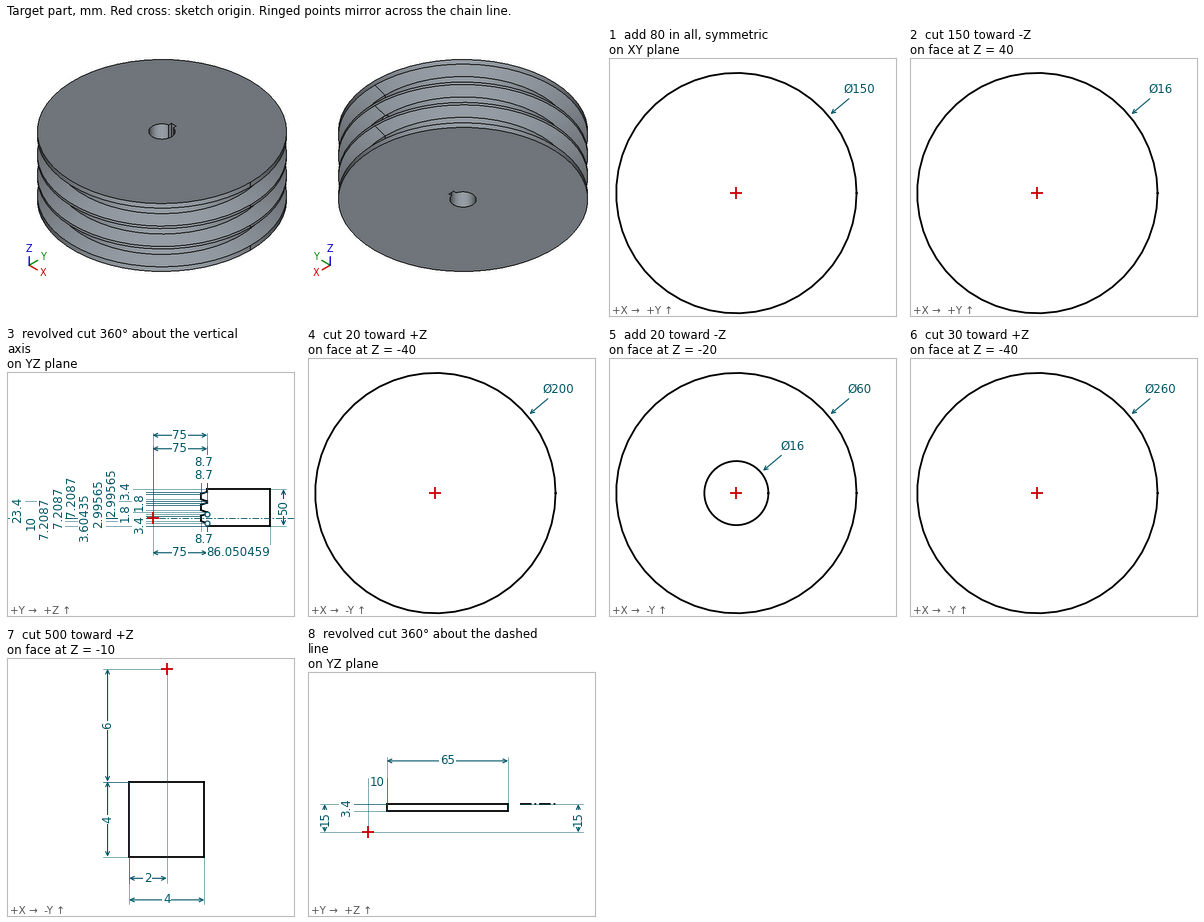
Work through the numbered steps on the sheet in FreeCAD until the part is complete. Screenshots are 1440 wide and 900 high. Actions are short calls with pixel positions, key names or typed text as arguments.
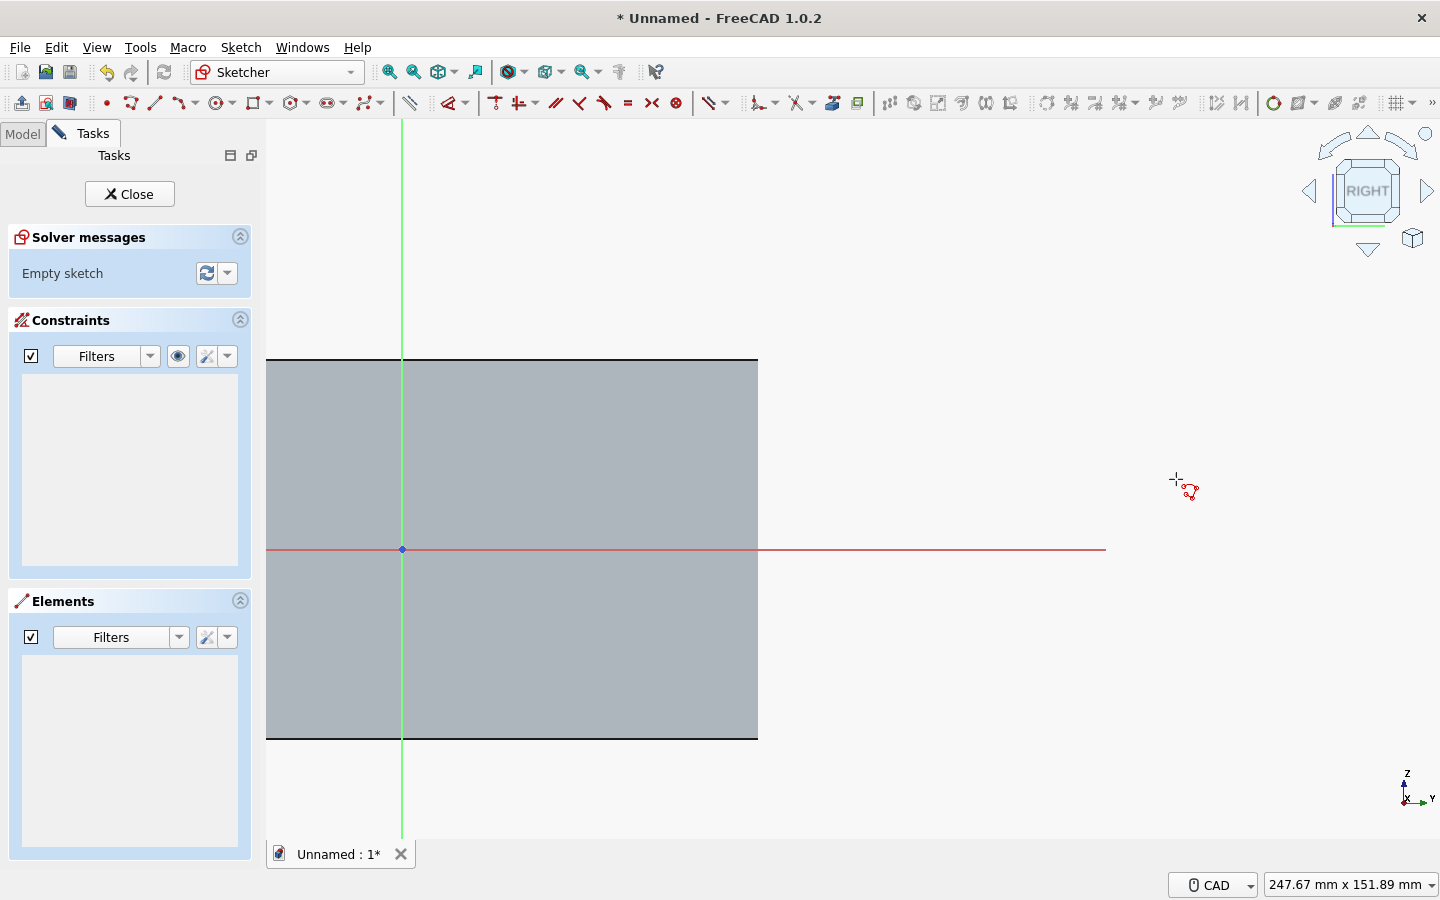
click(716, 533)
click(716, 567)
click(758, 581)
click(758, 597)
click(1166, 597)
click(1166, 360)
click(758, 360)
click(758, 376)
click(716, 391)
click(716, 425)
click(758, 439)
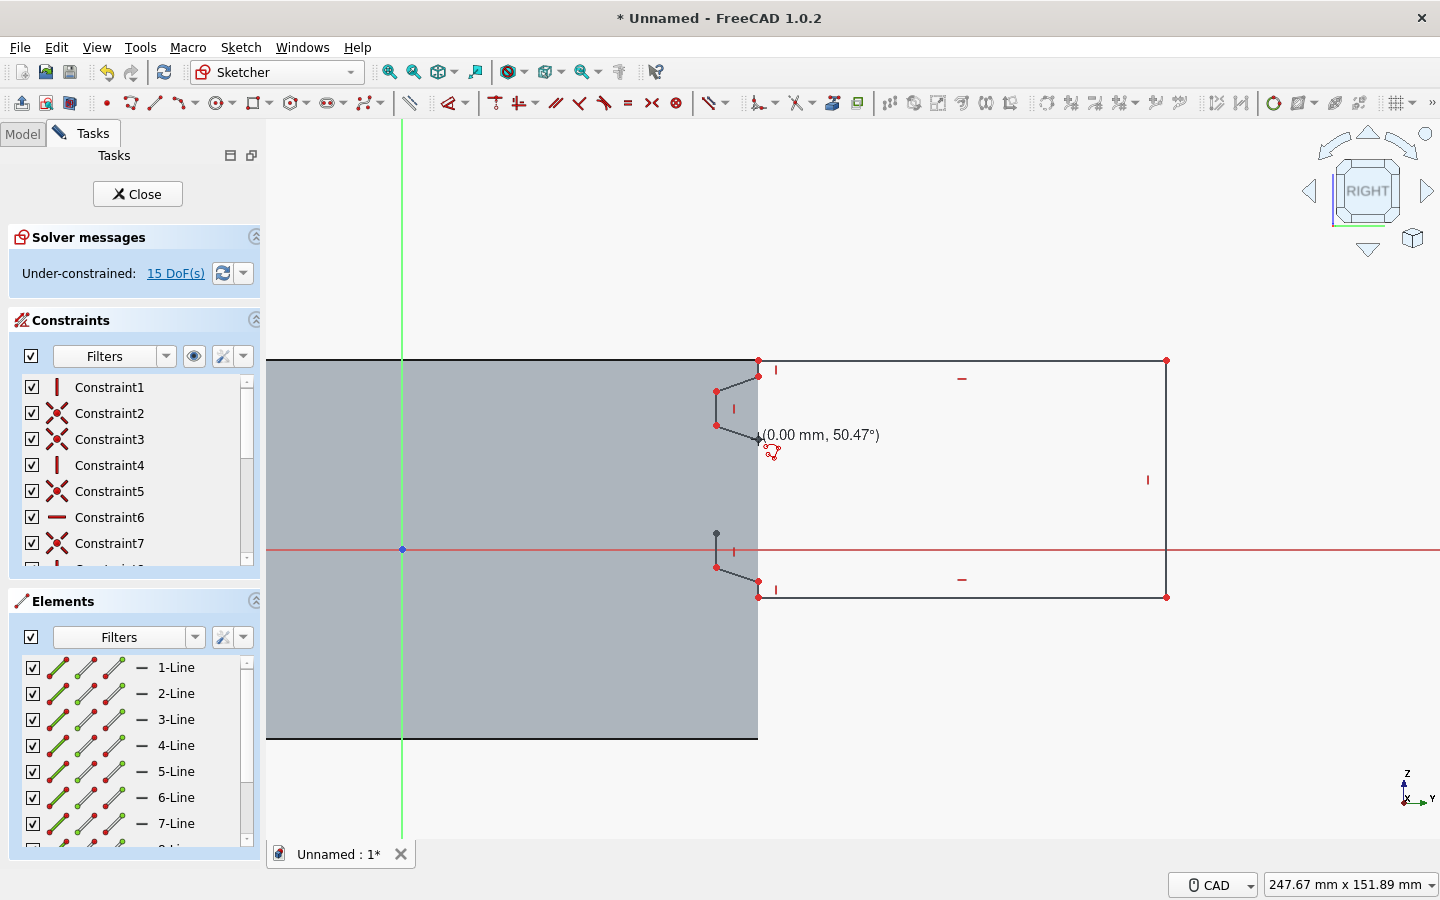
scroll(758, 447, up, 4)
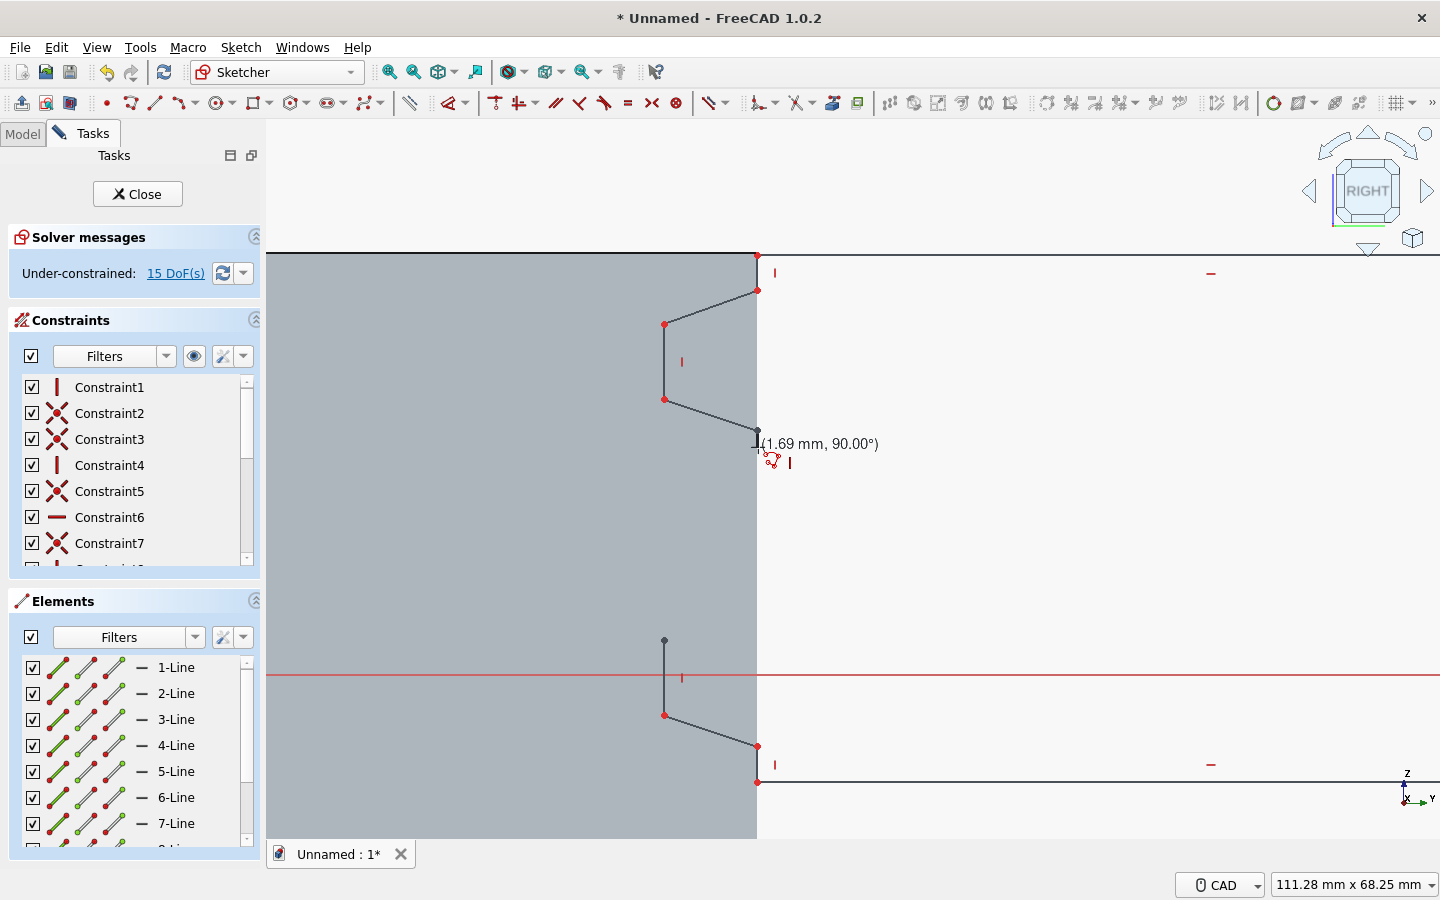
click(757, 448)
click(665, 479)
click(665, 555)
click(757, 587)
click(757, 606)
click(664, 640)
key(Escape)
key(Escape)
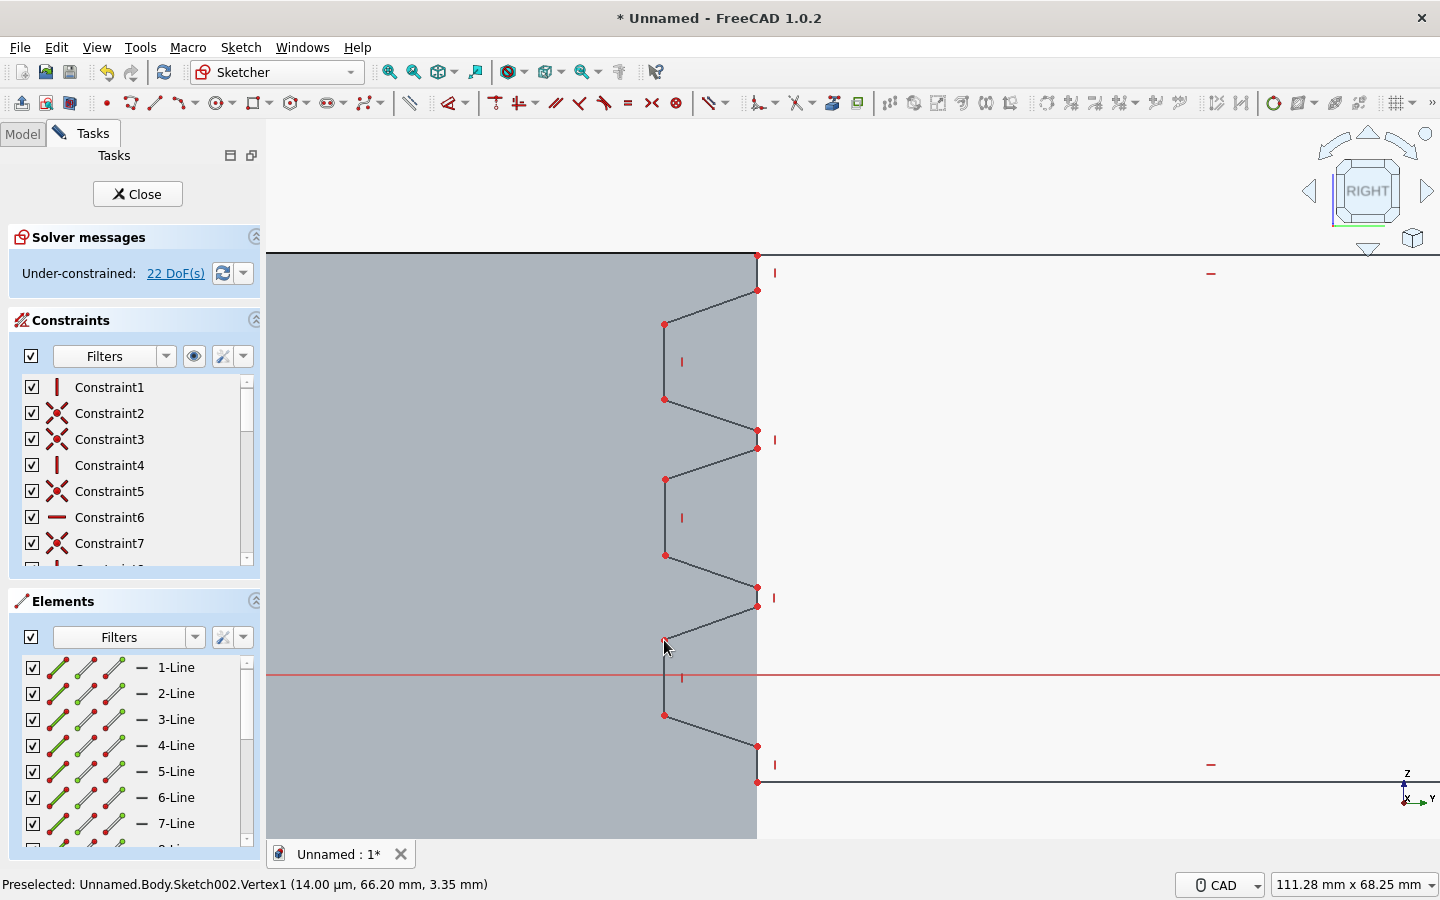
click(757, 747)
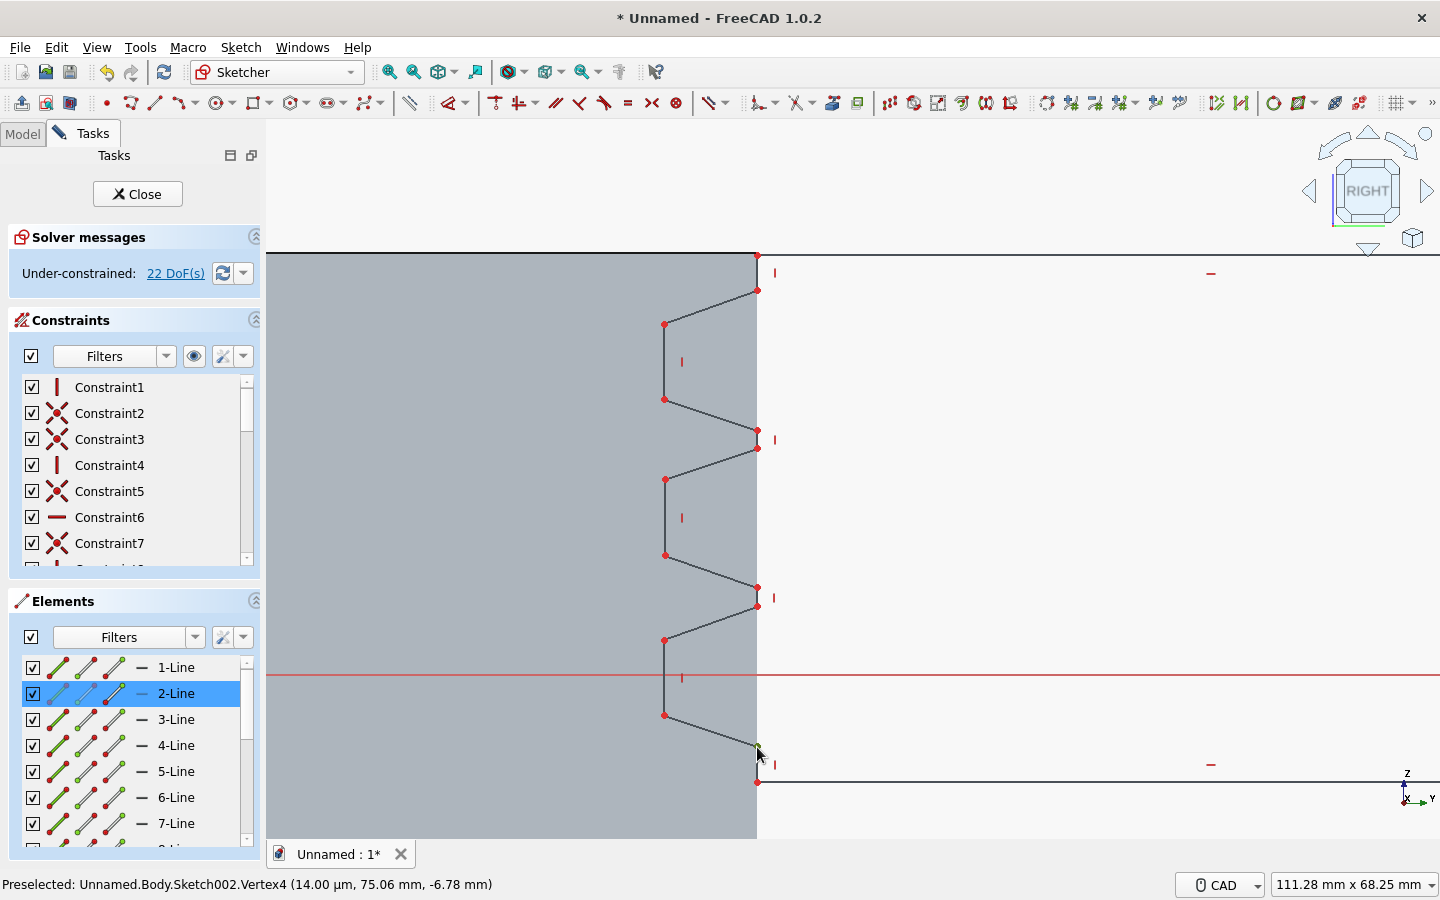
click(757, 607)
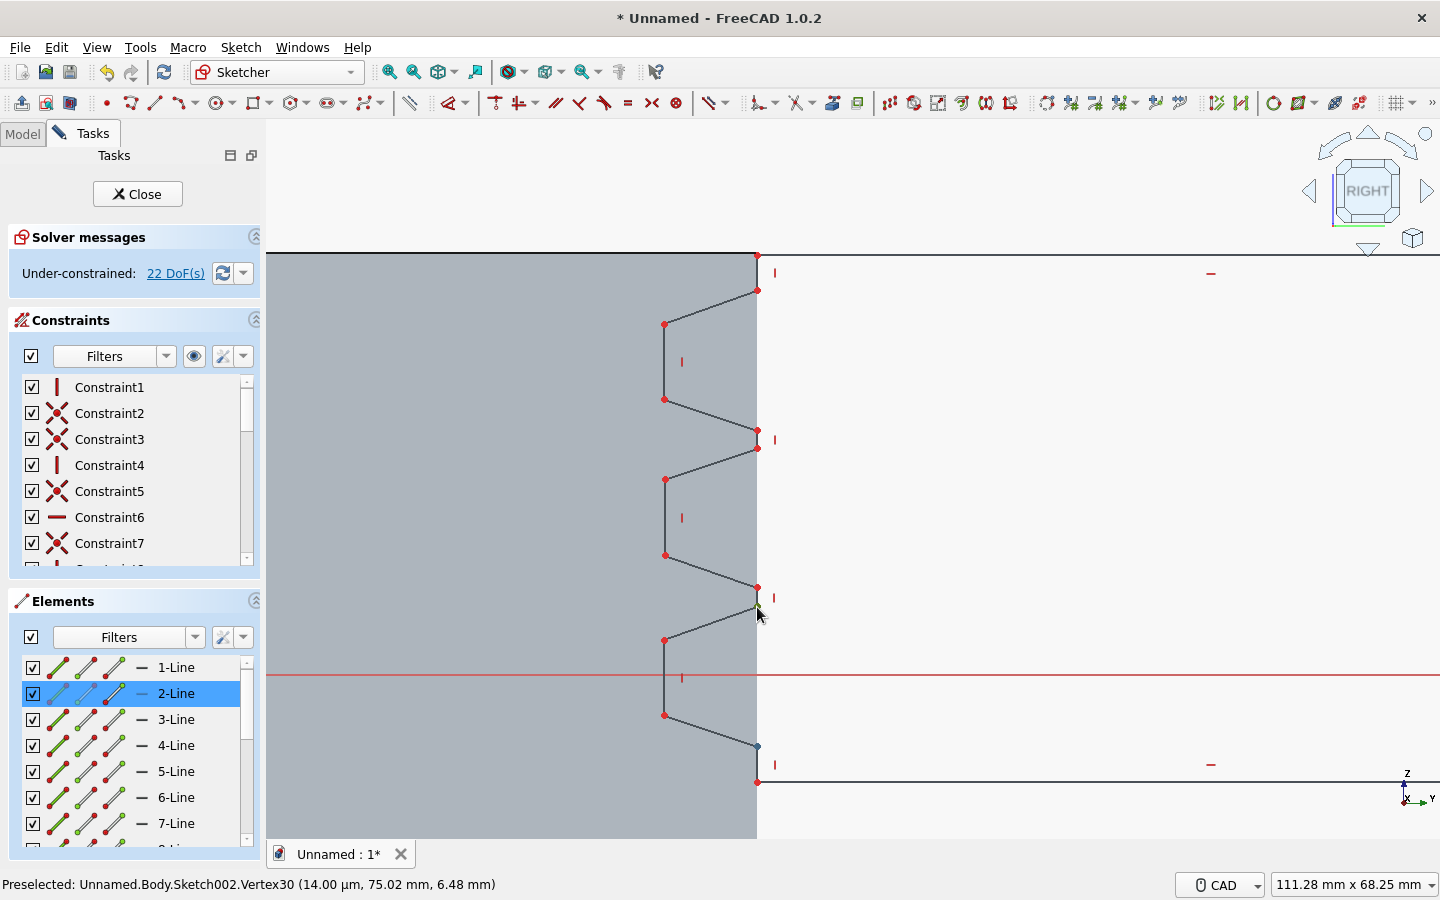
click(364, 675)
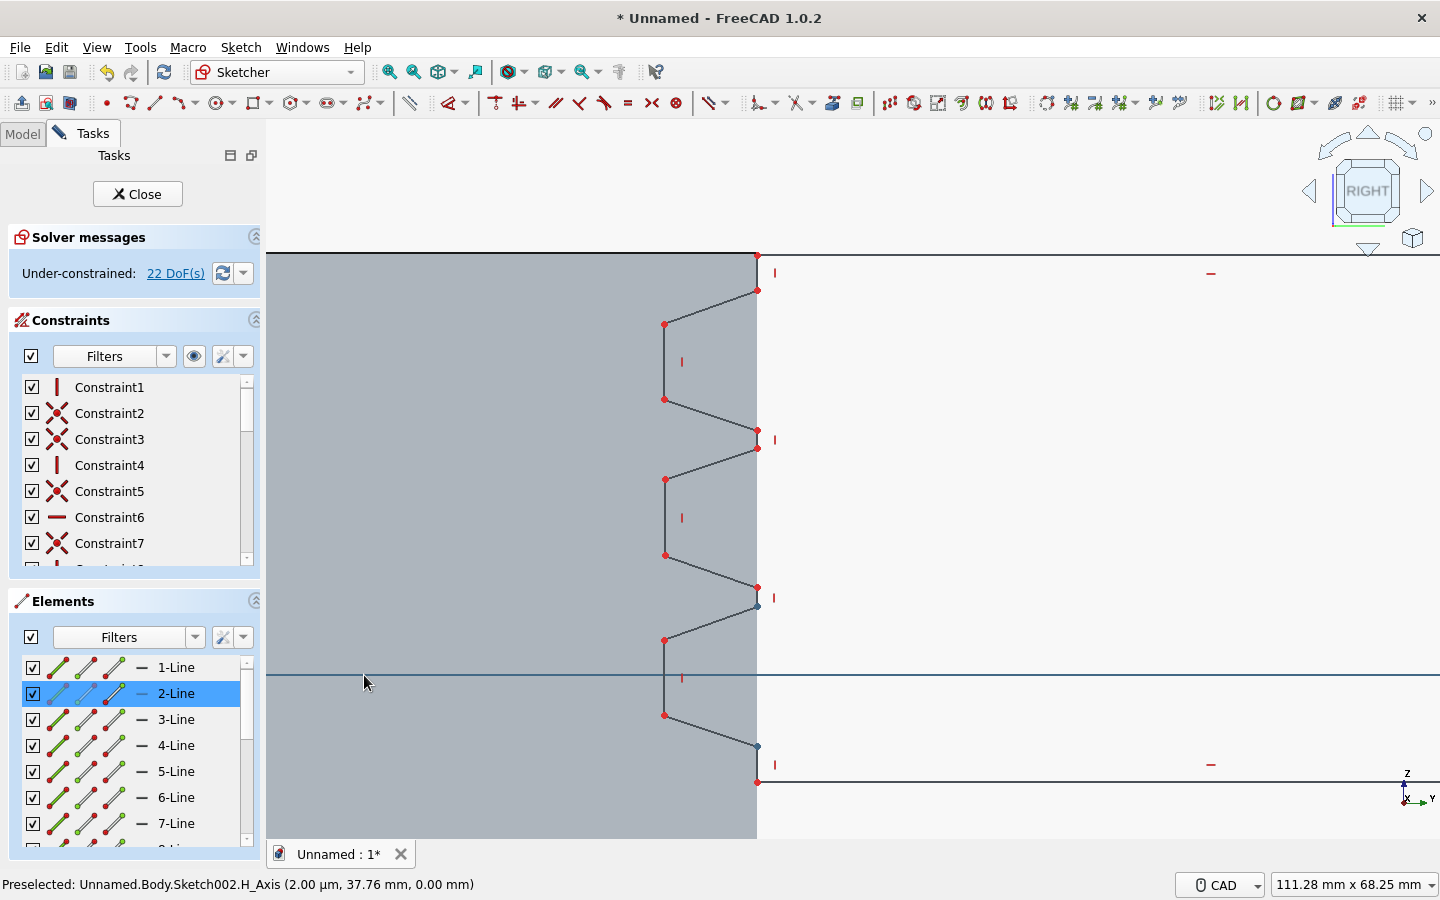
click(652, 104)